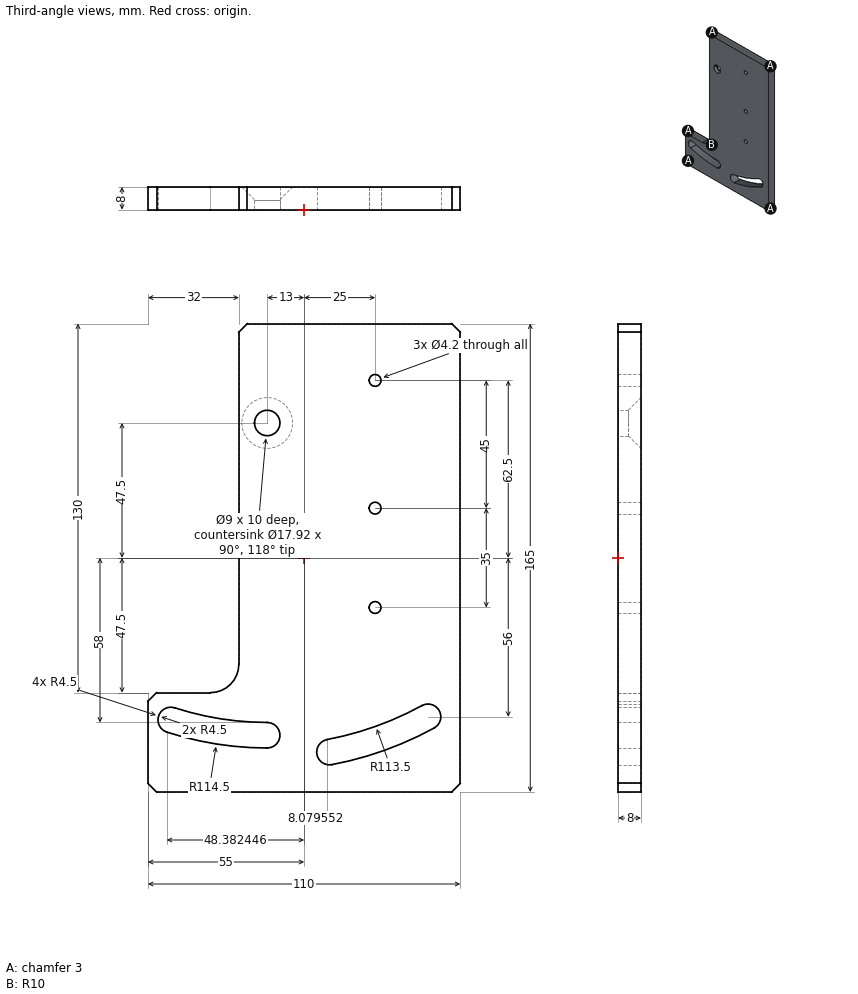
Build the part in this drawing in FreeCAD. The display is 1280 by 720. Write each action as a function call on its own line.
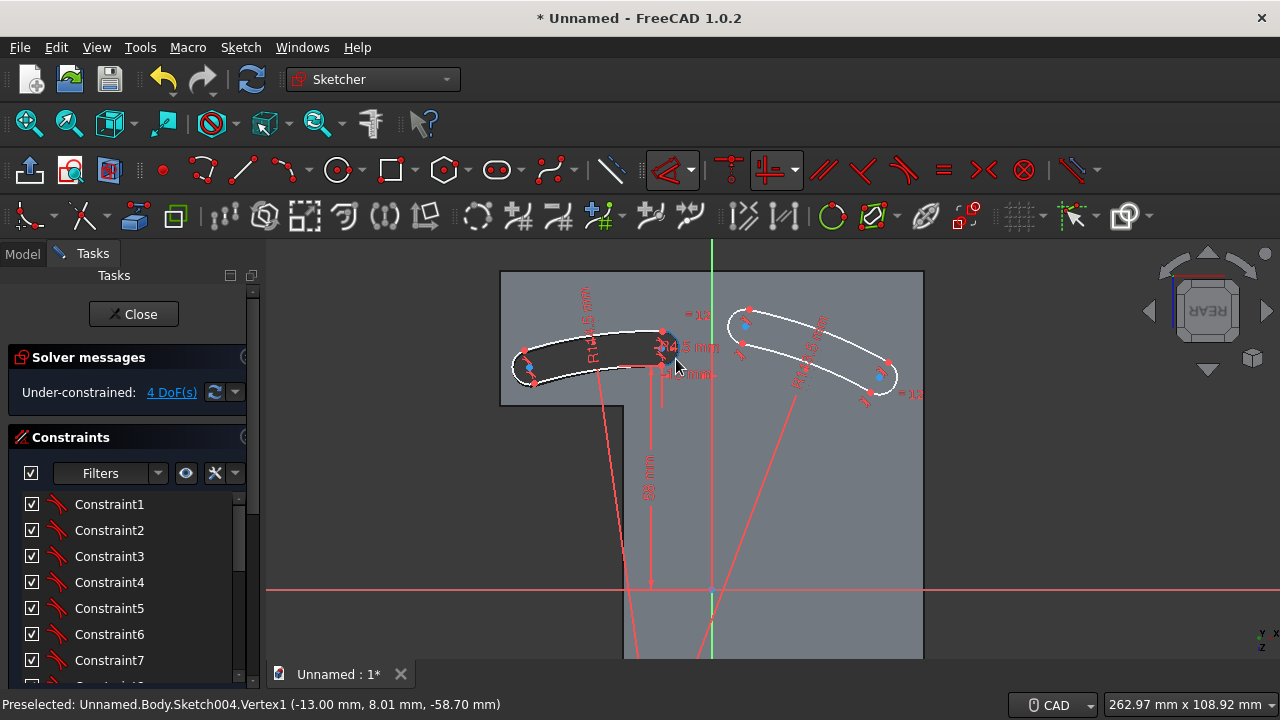
scroll(704, 338, down, 3)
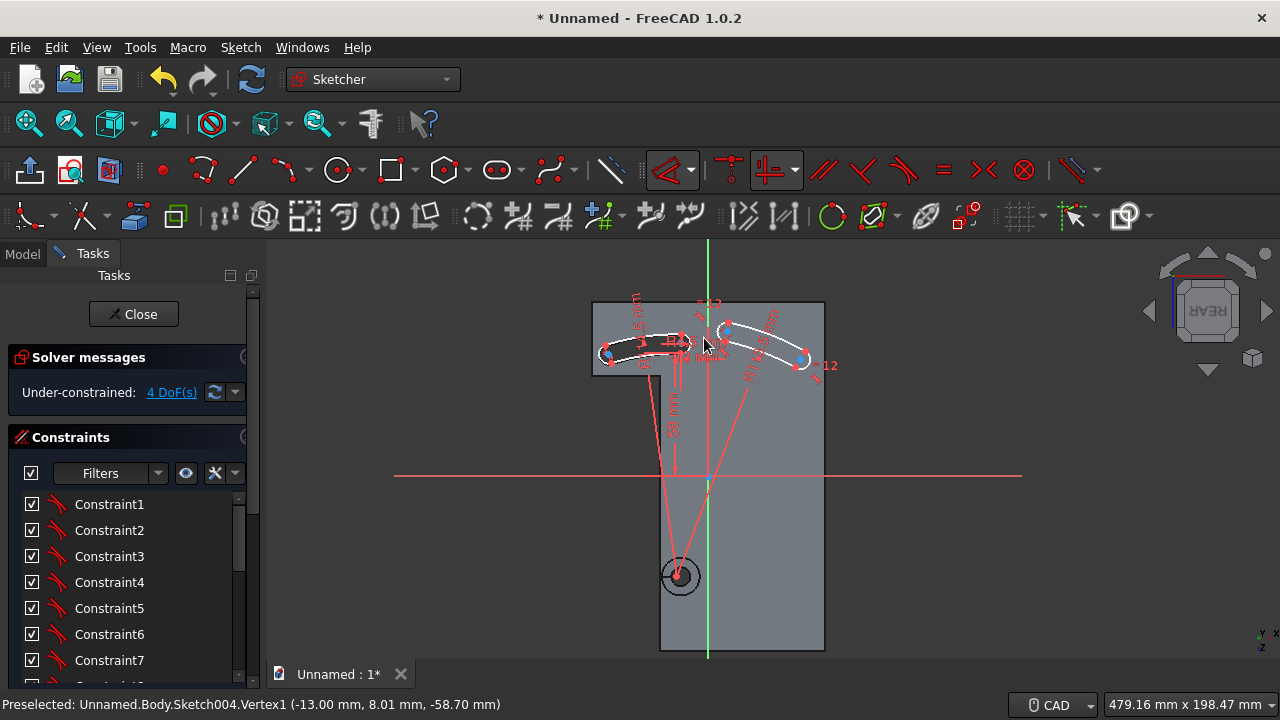
scroll(677, 577, up, 2)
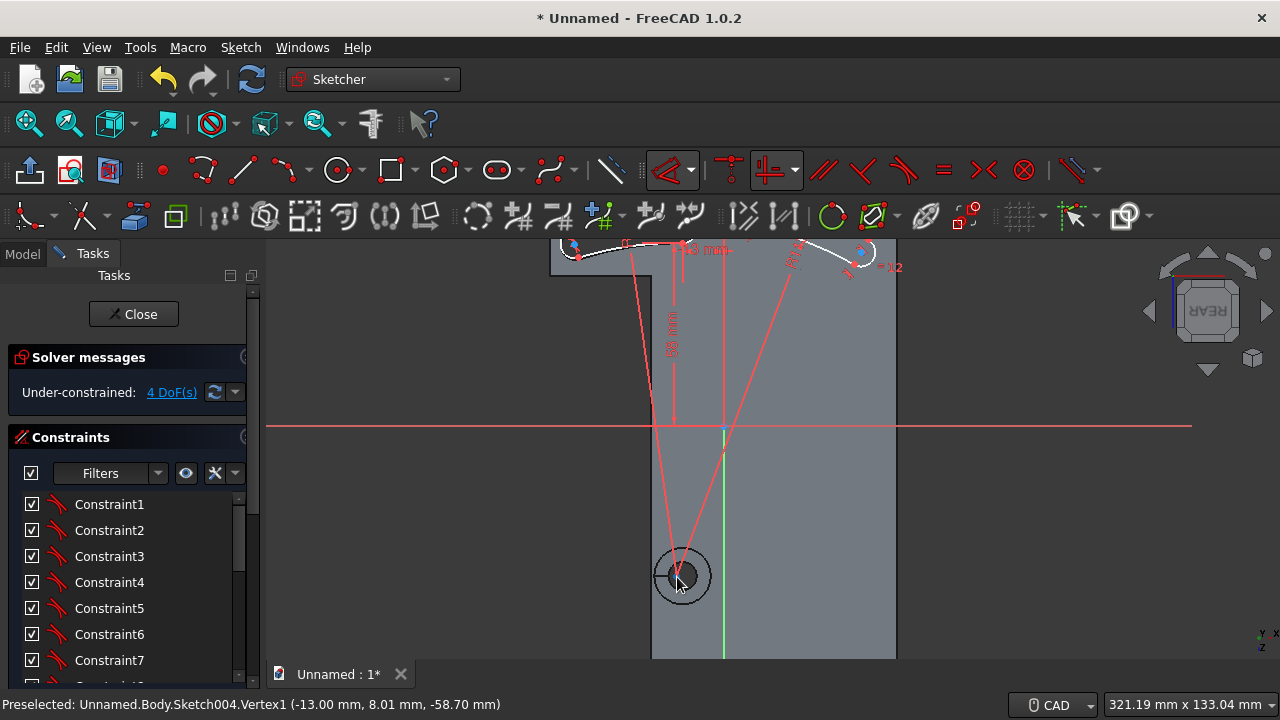
click(677, 576)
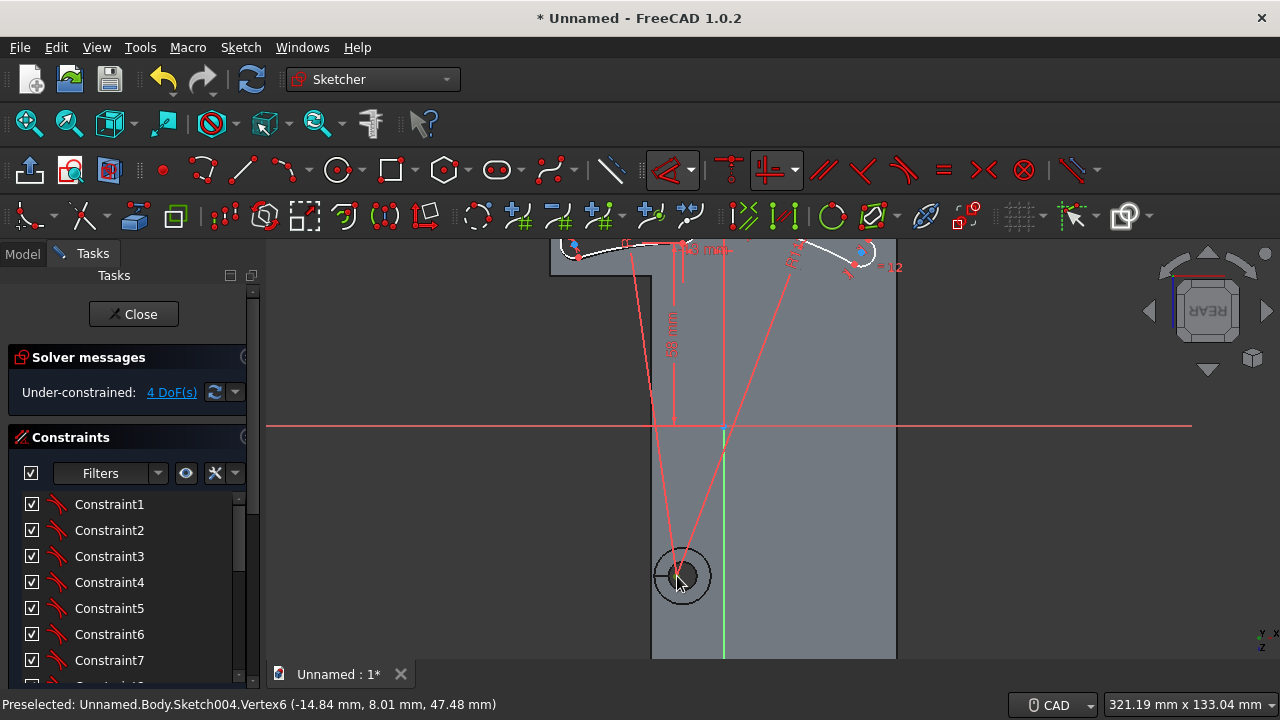
click(694, 170)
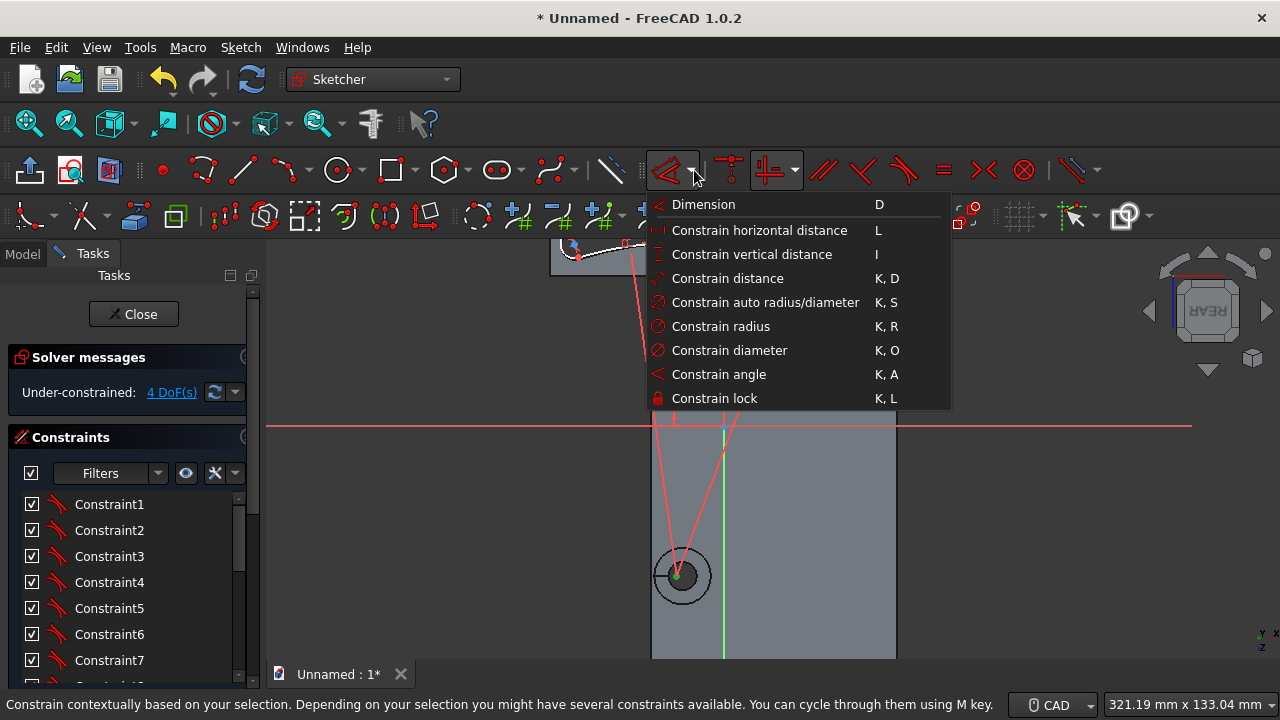
click(799, 230)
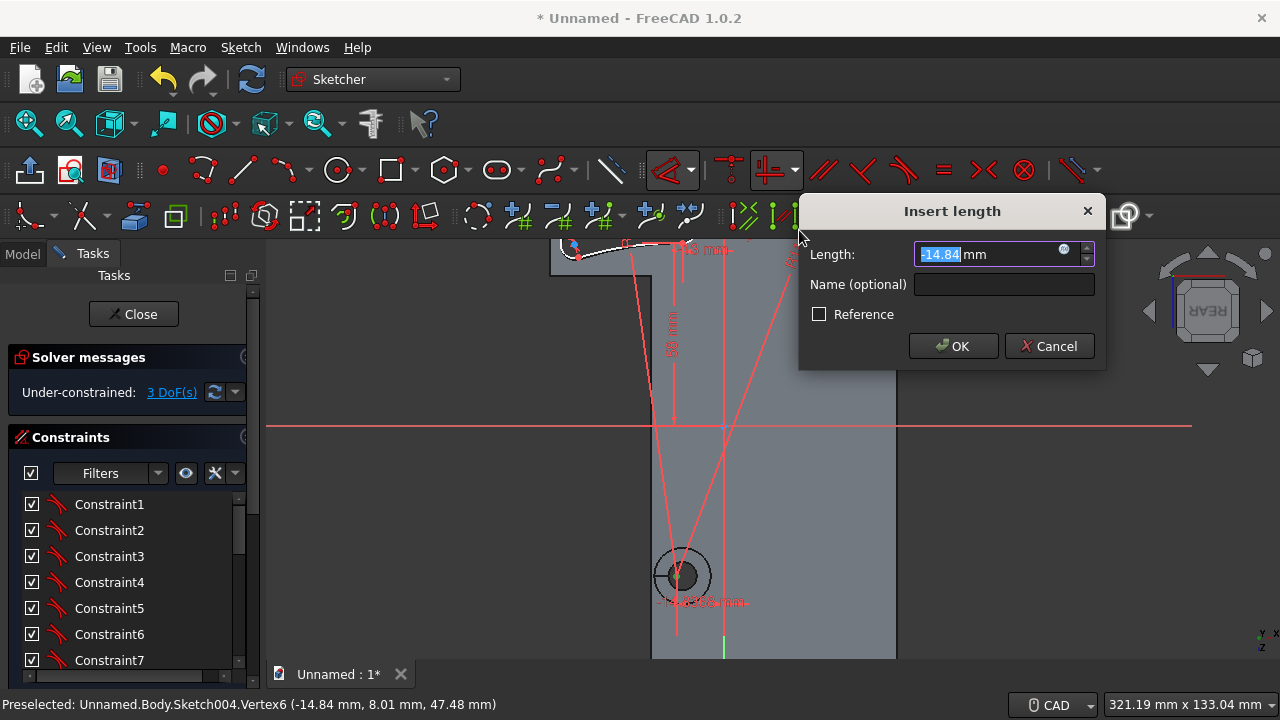
text(-13)
key(Return)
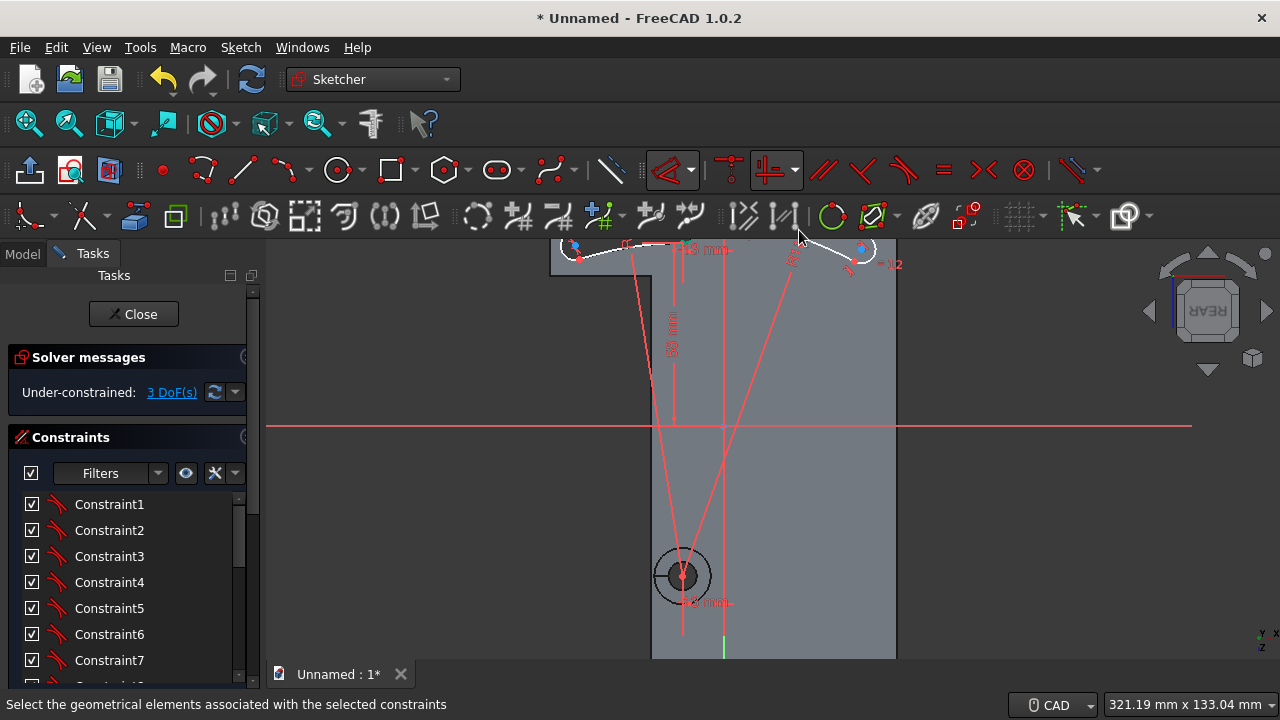
scroll(677, 631, down, 2)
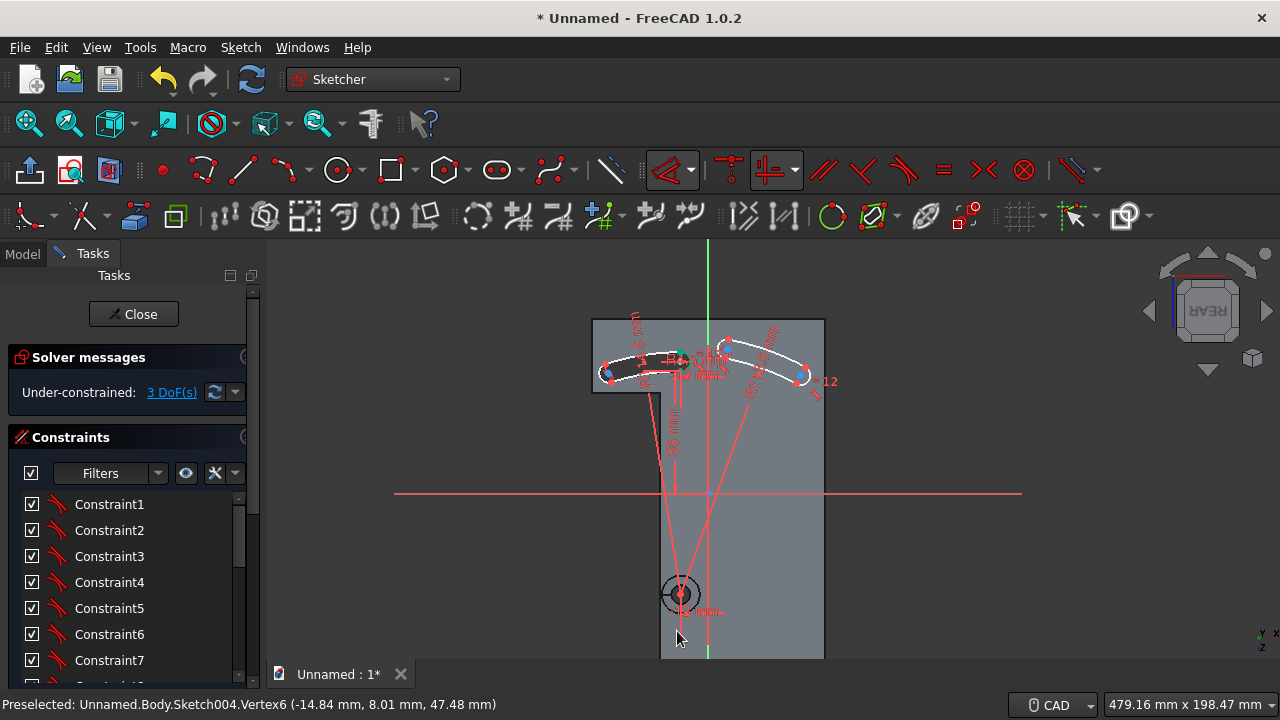
scroll(705, 378, up, 3)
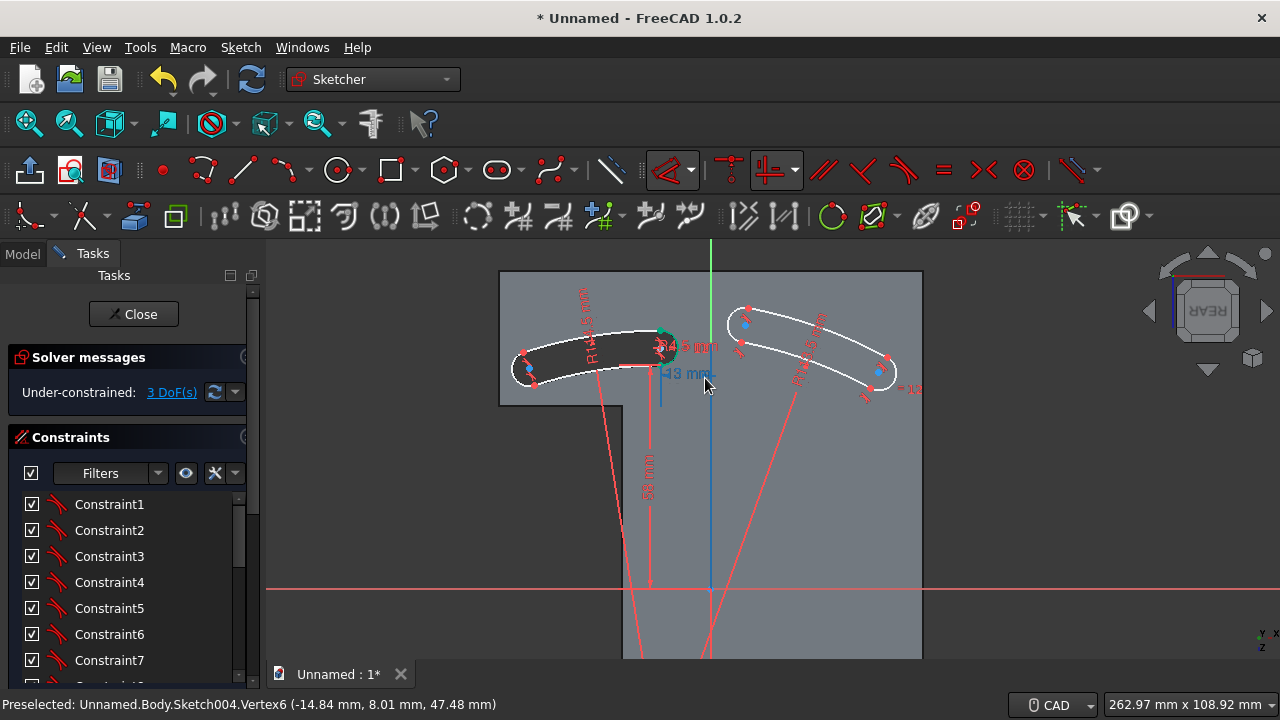
click(879, 373)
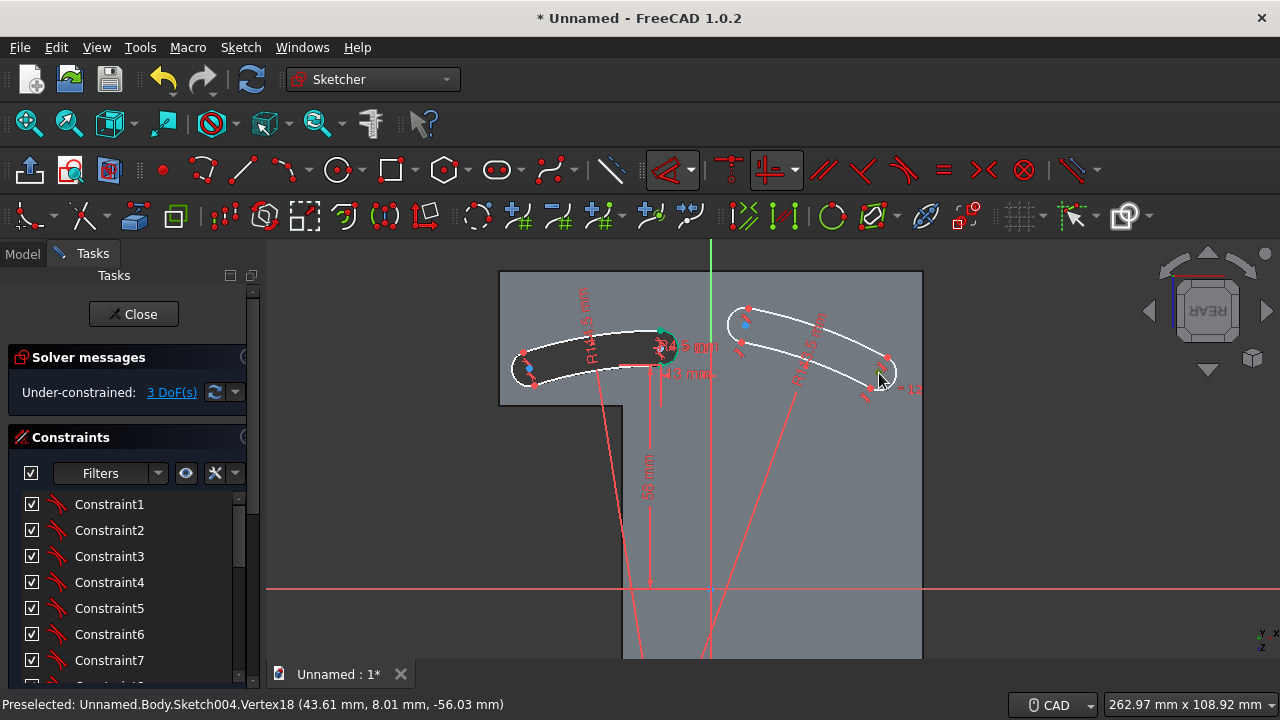
key(i)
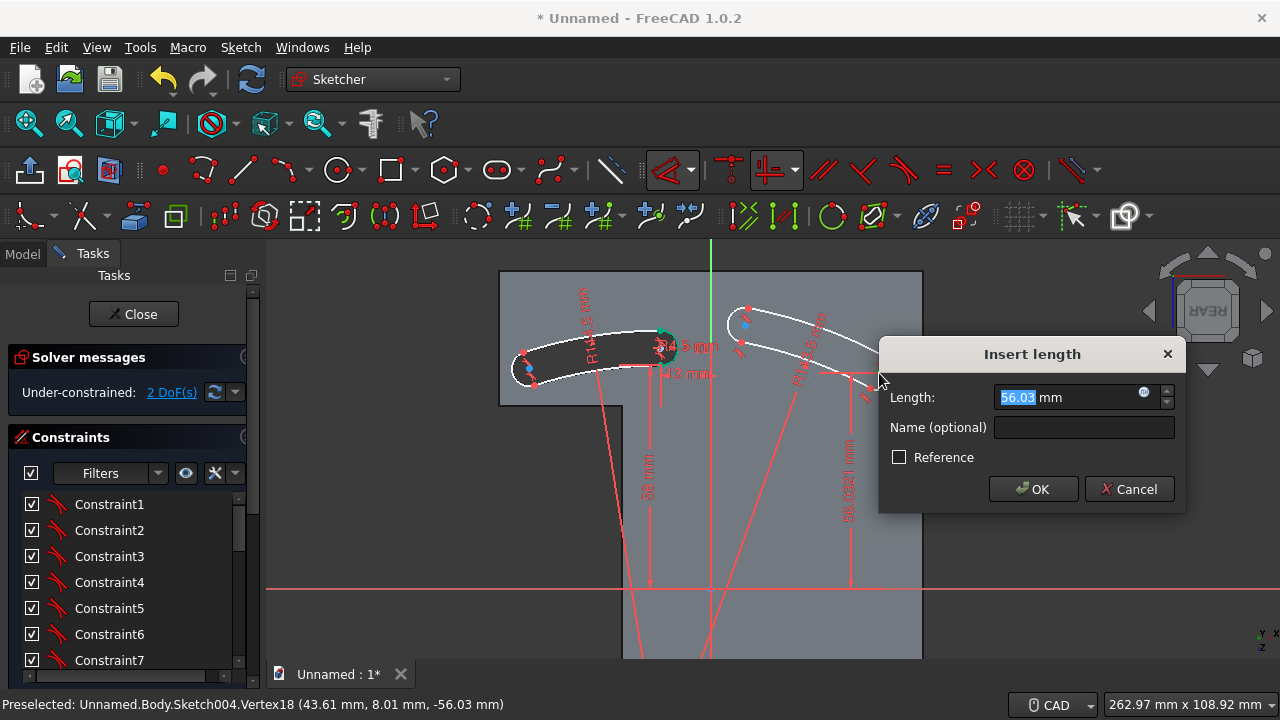
text(56)
key(Return)